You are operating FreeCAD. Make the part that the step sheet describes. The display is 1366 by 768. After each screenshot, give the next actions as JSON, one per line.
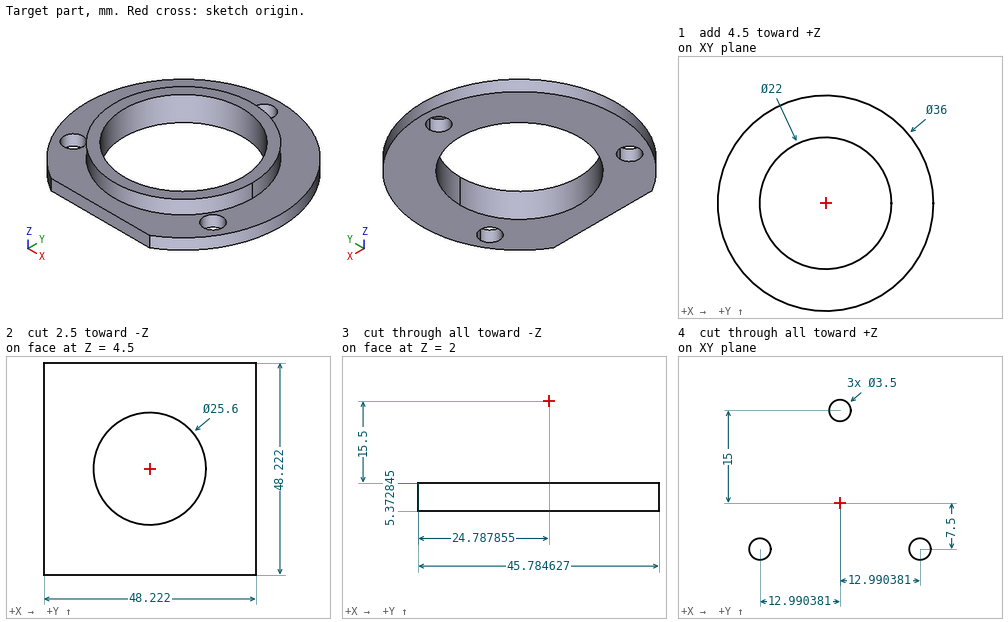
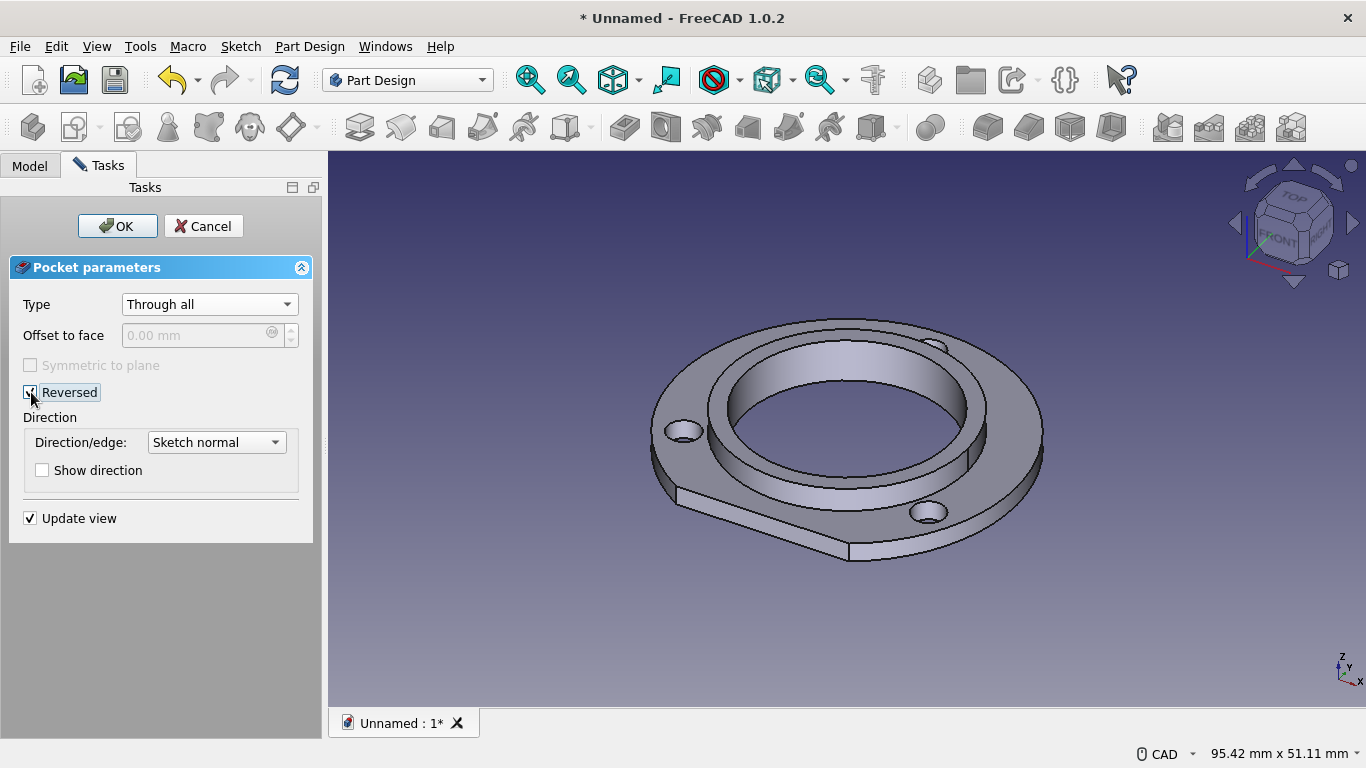
{"action": "left_click", "coordinate": [118, 226]}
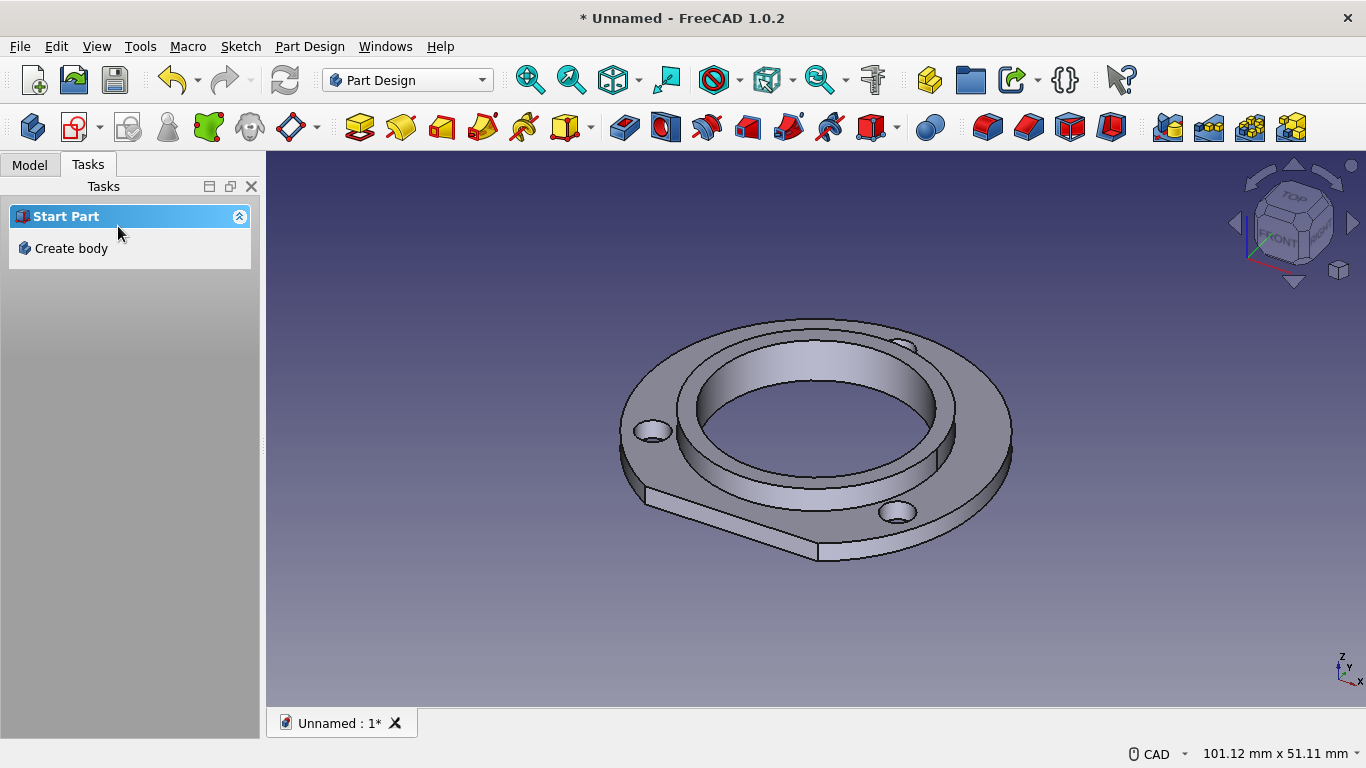
{"action": "key", "text": "0"}